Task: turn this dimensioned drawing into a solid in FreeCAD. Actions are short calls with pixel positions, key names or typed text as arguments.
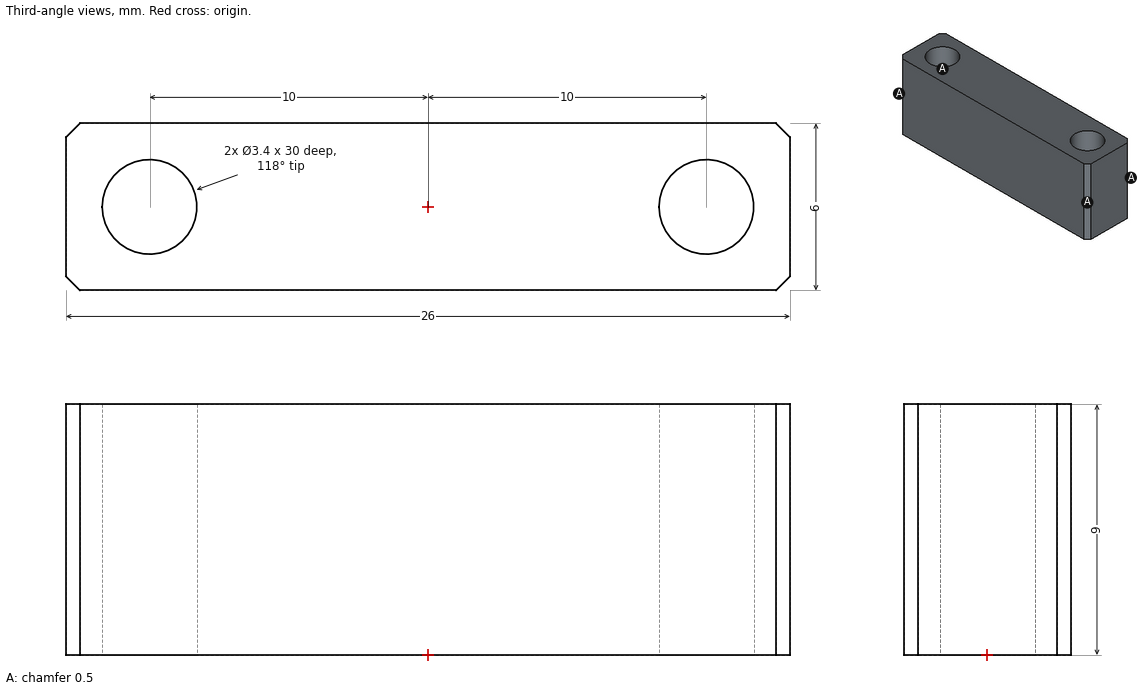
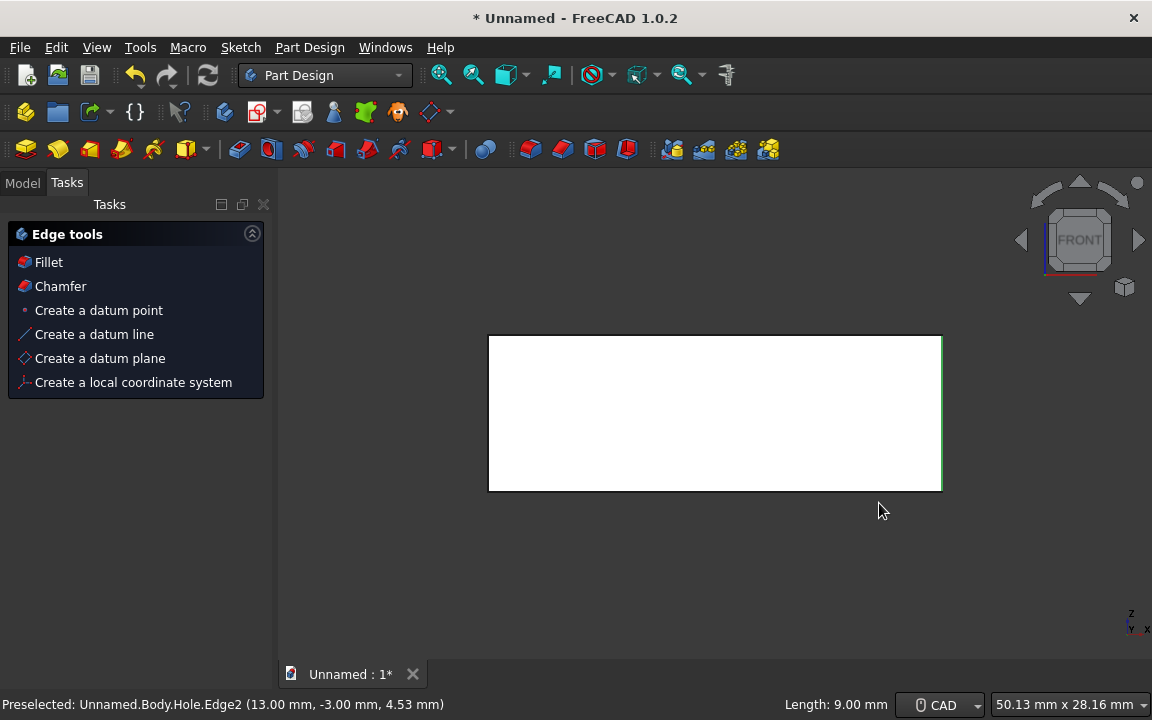
click(488, 412, ctrl)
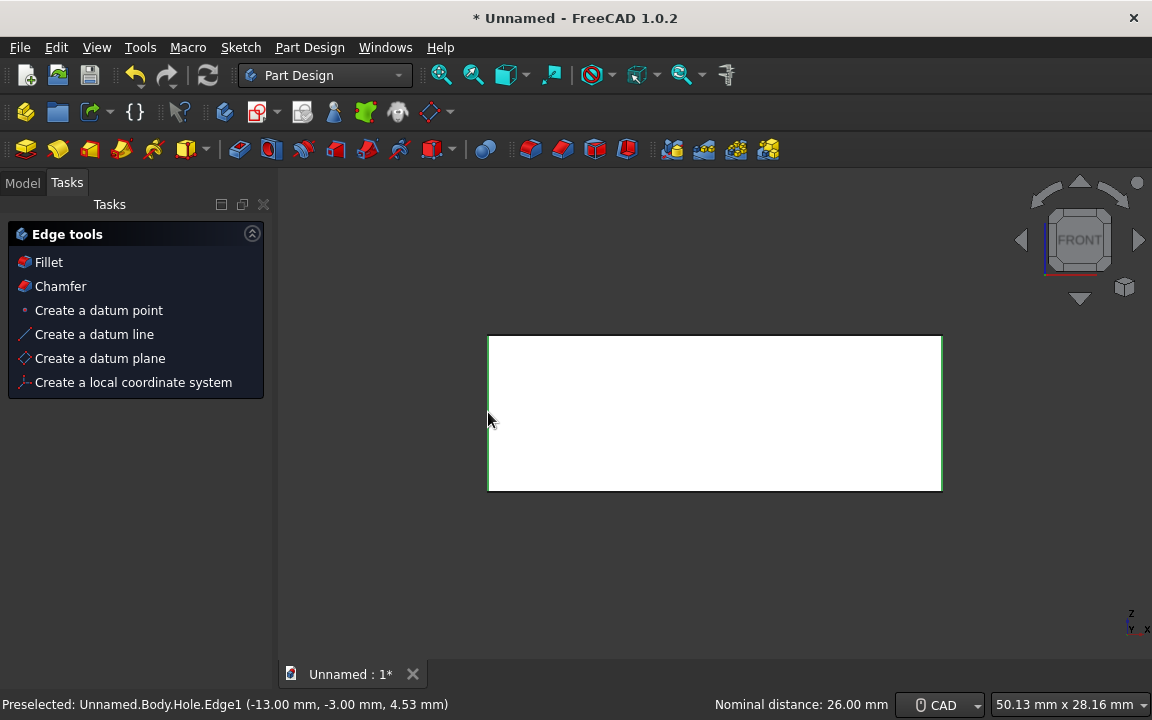
key(3)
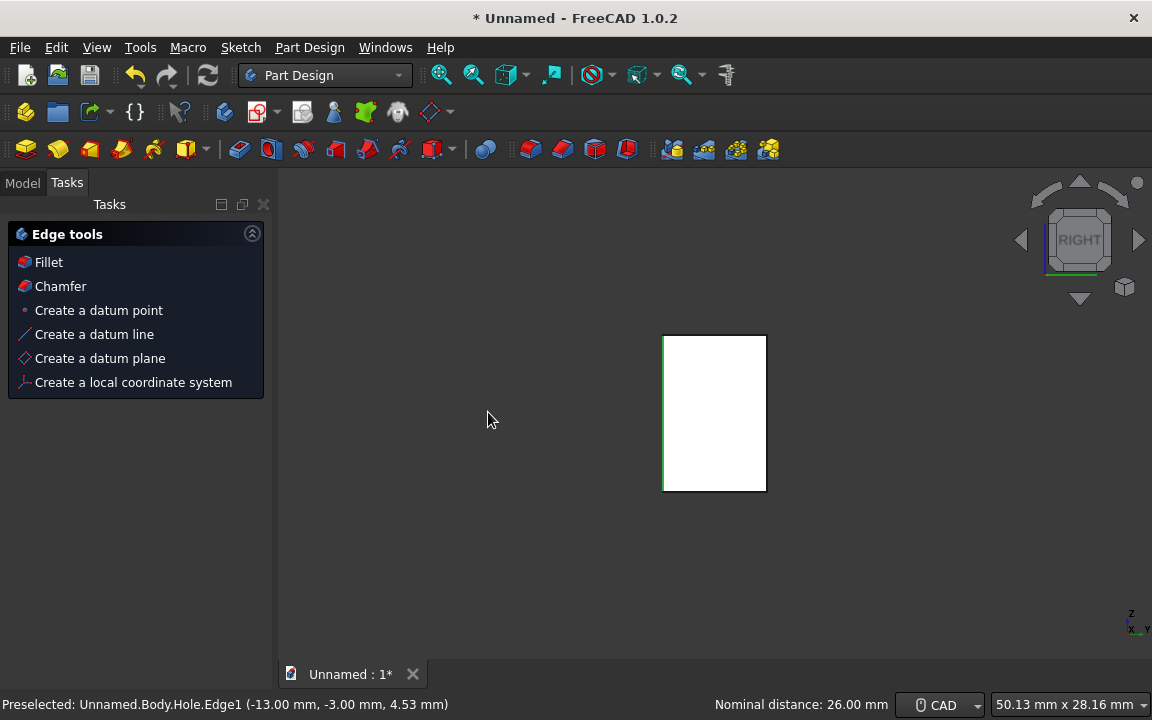
key(v)
key(f)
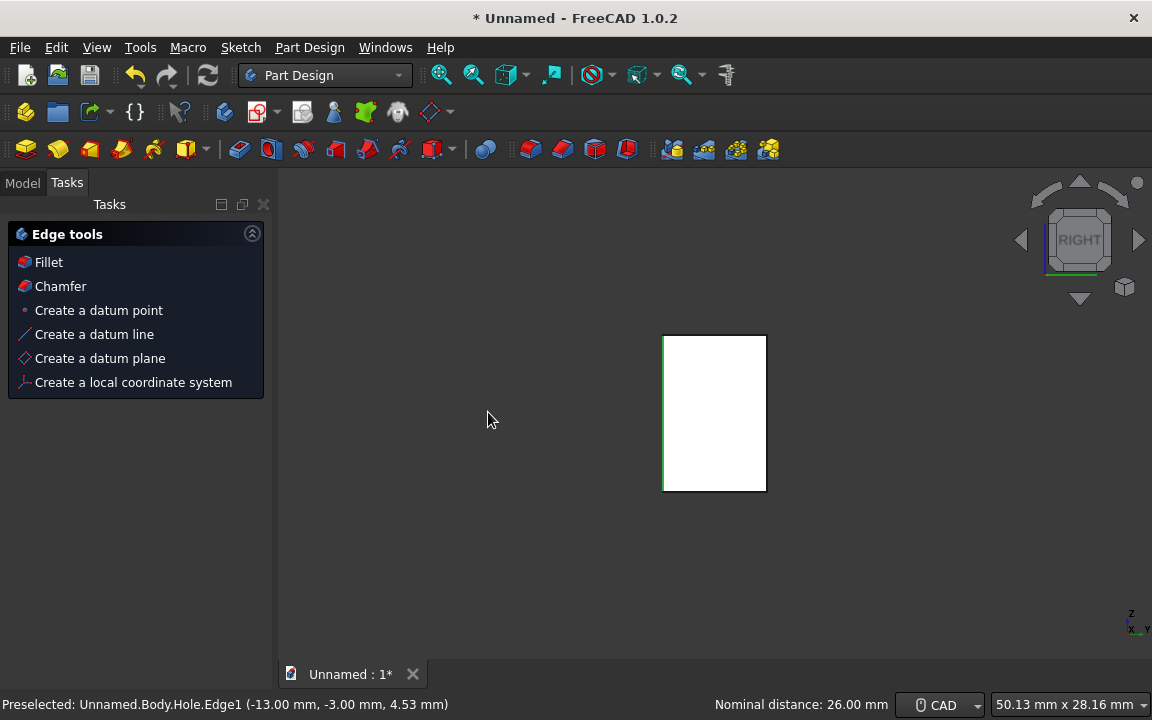
click(767, 412, ctrl)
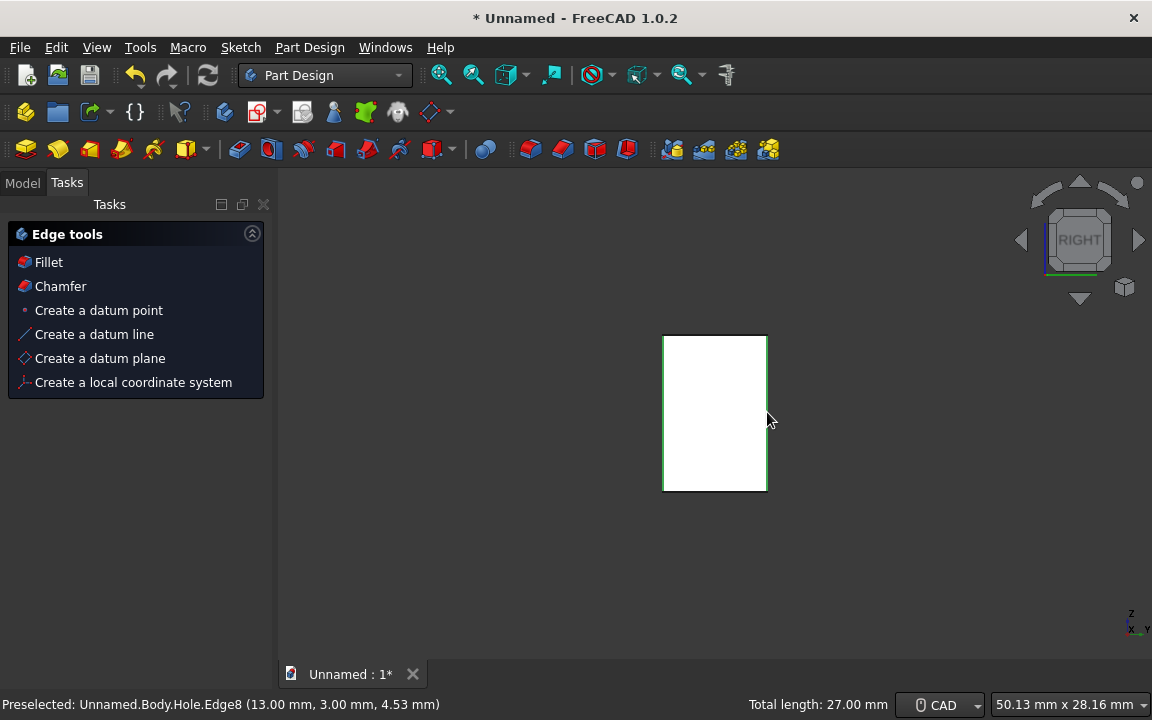
key(5)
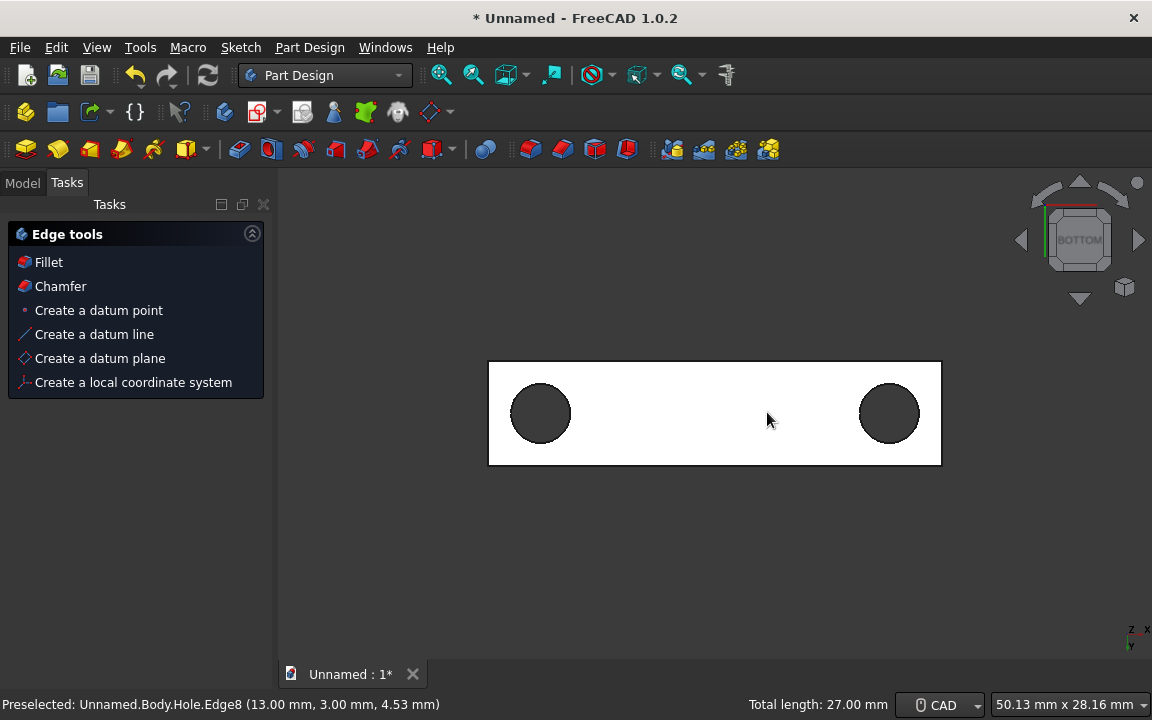
key(4)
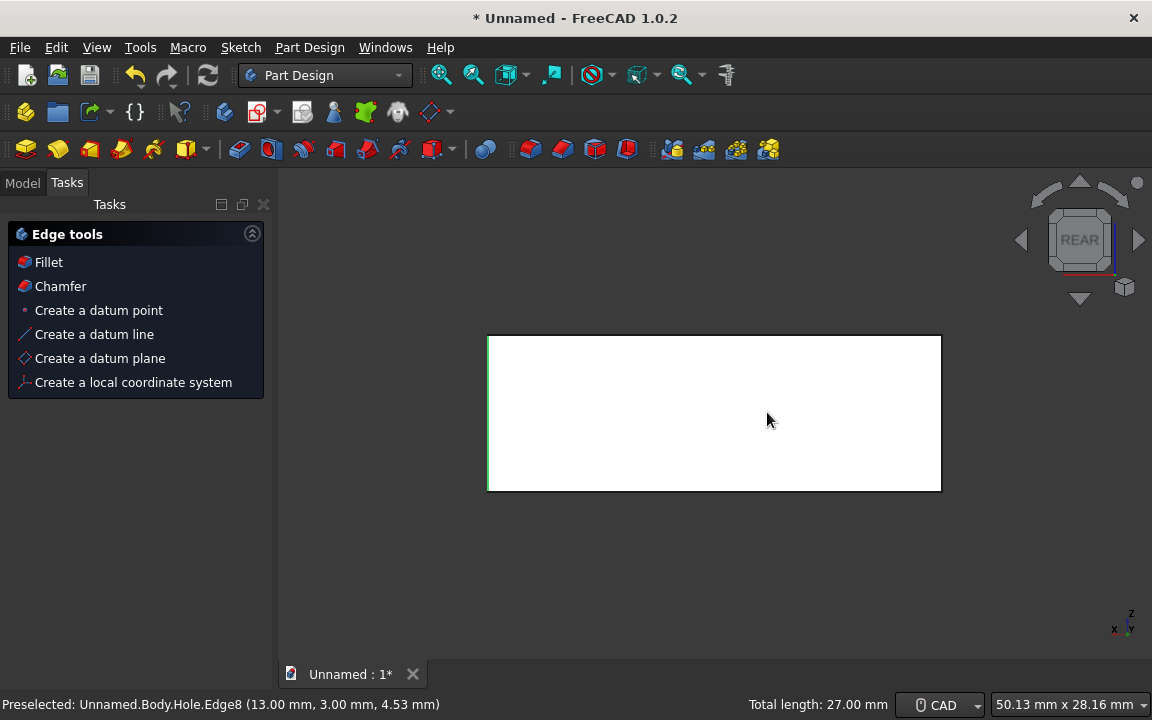
click(942, 412, ctrl)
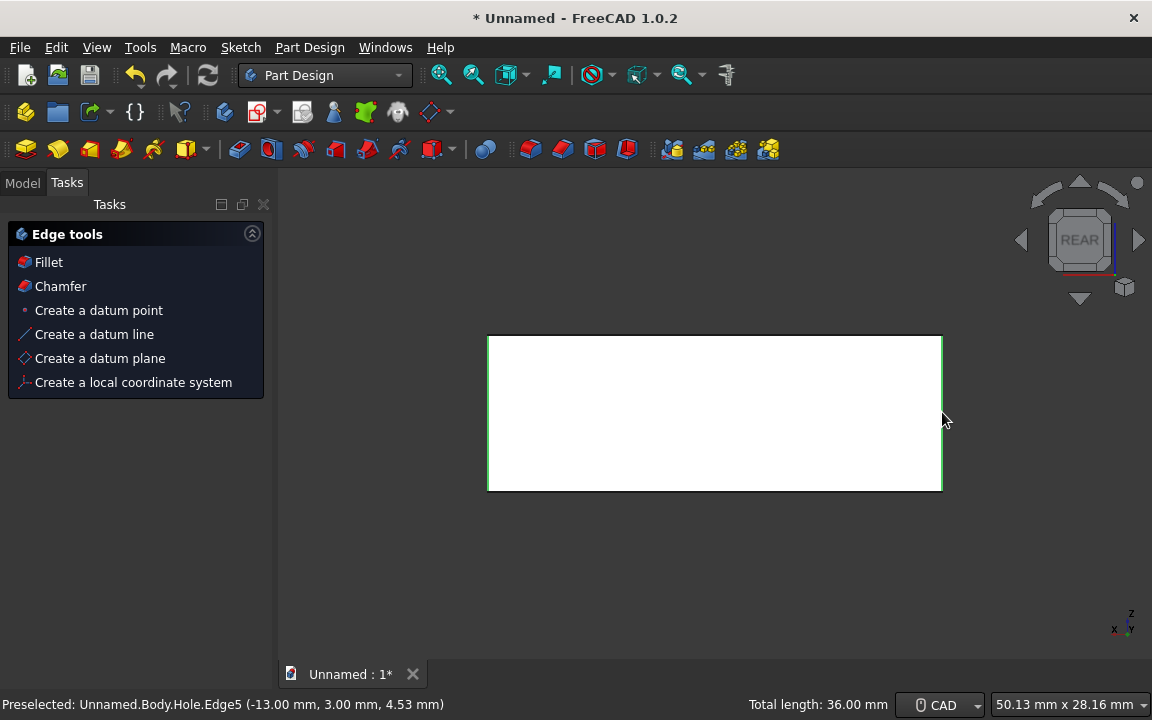
click(564, 150)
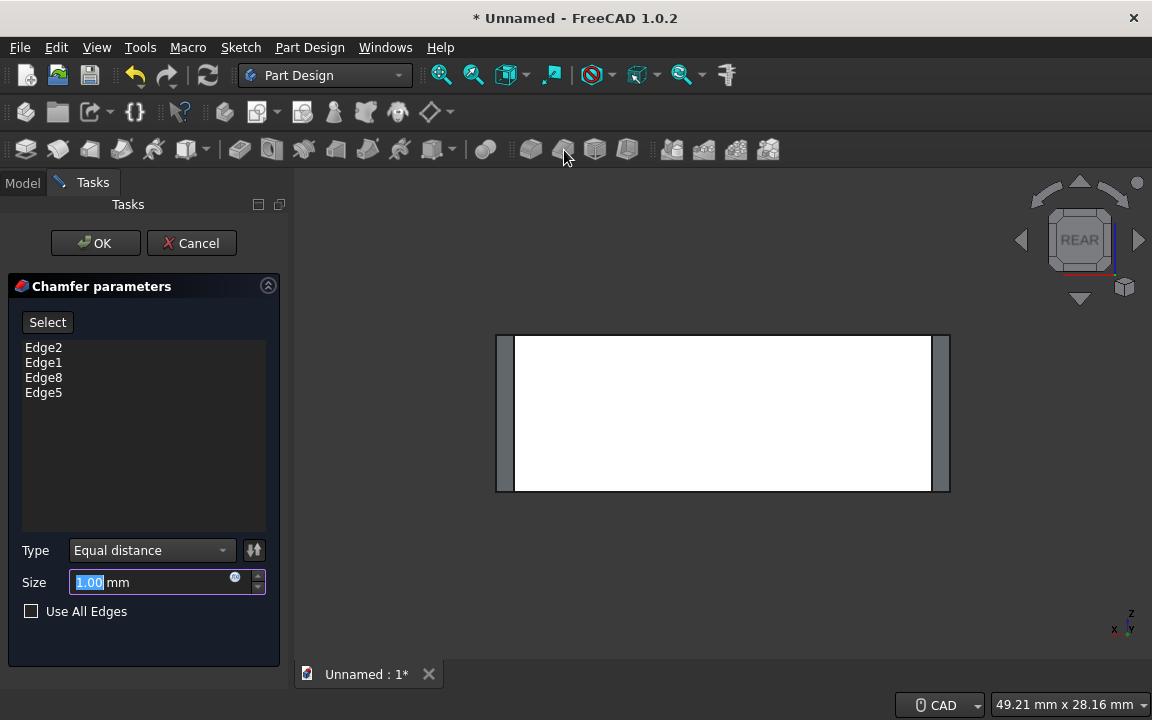
text(0.5)
key(Tab)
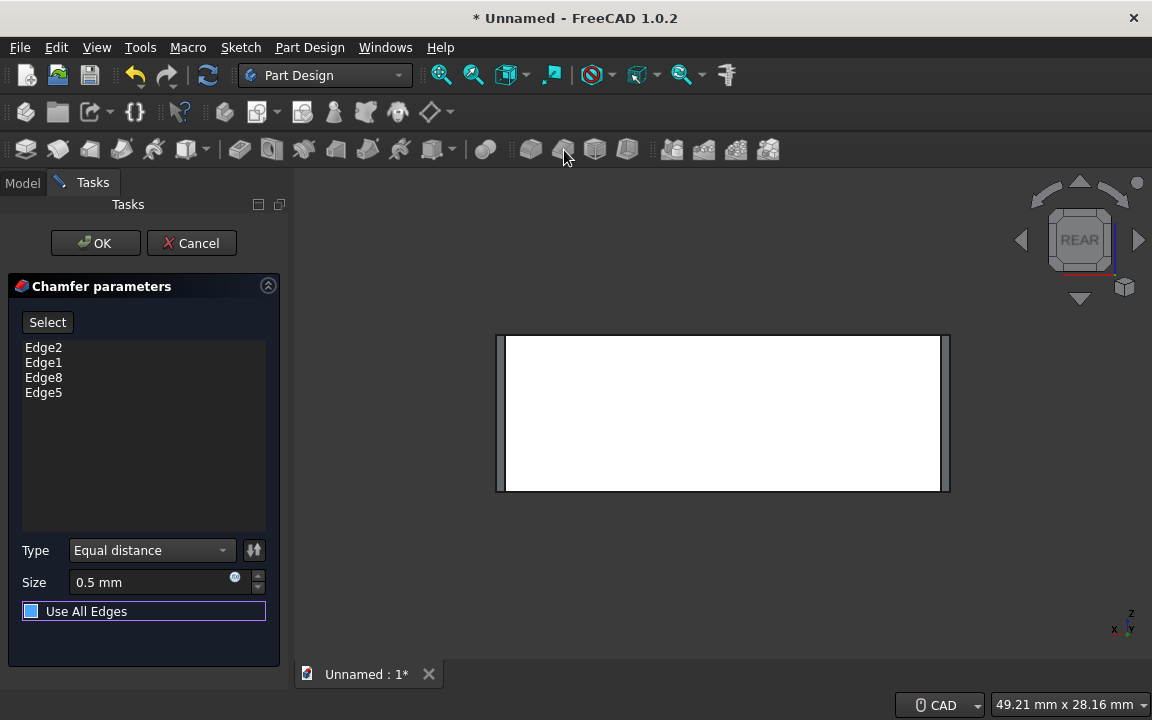
click(96, 243)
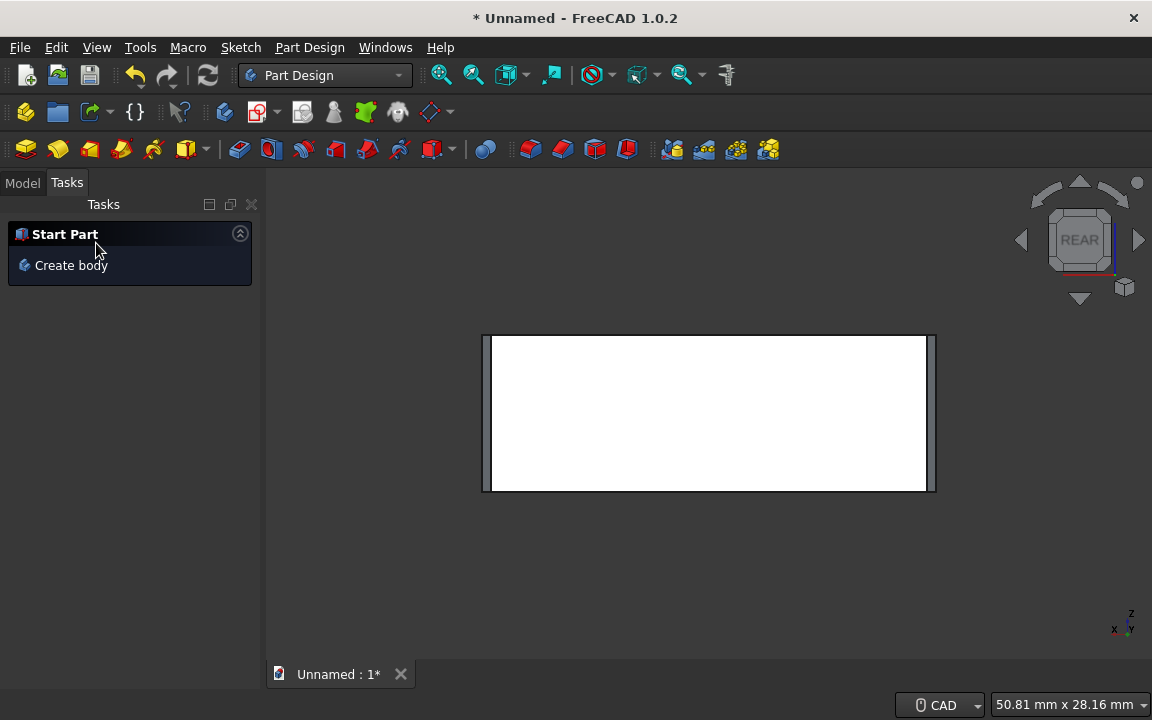
key(0)